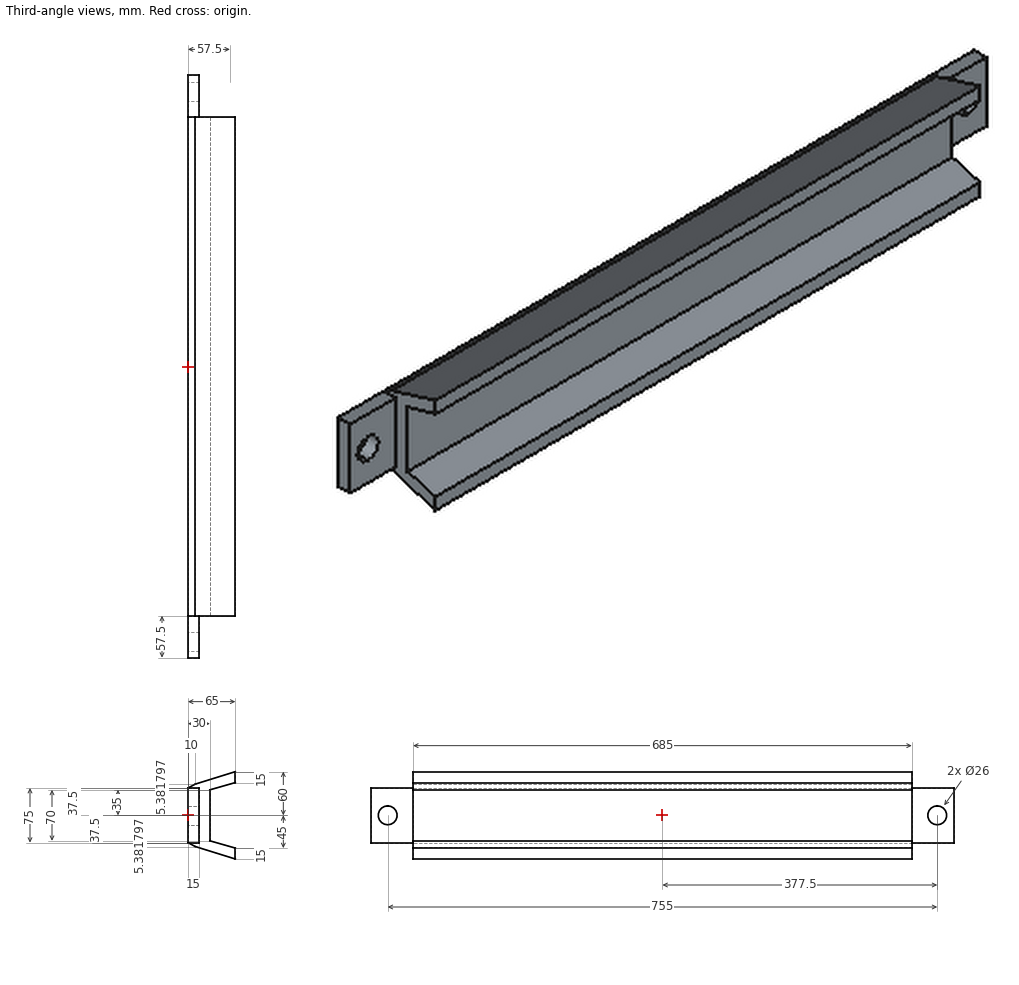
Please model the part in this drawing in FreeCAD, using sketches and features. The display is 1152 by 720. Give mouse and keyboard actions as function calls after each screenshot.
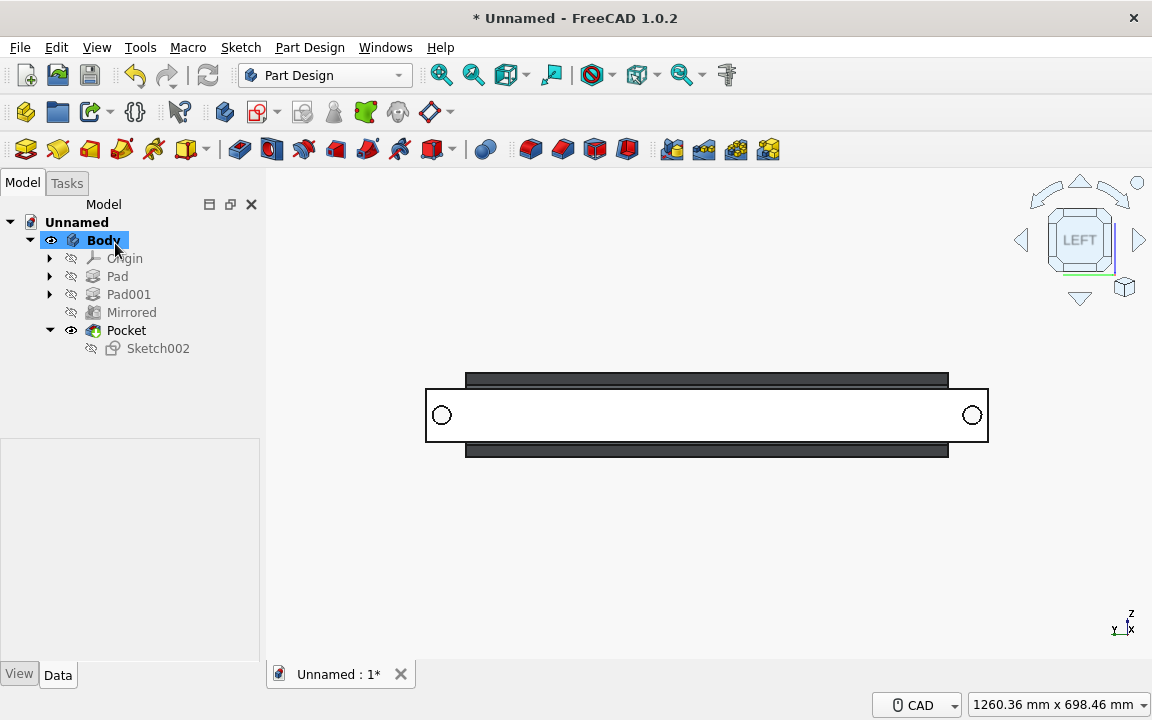
key(0)